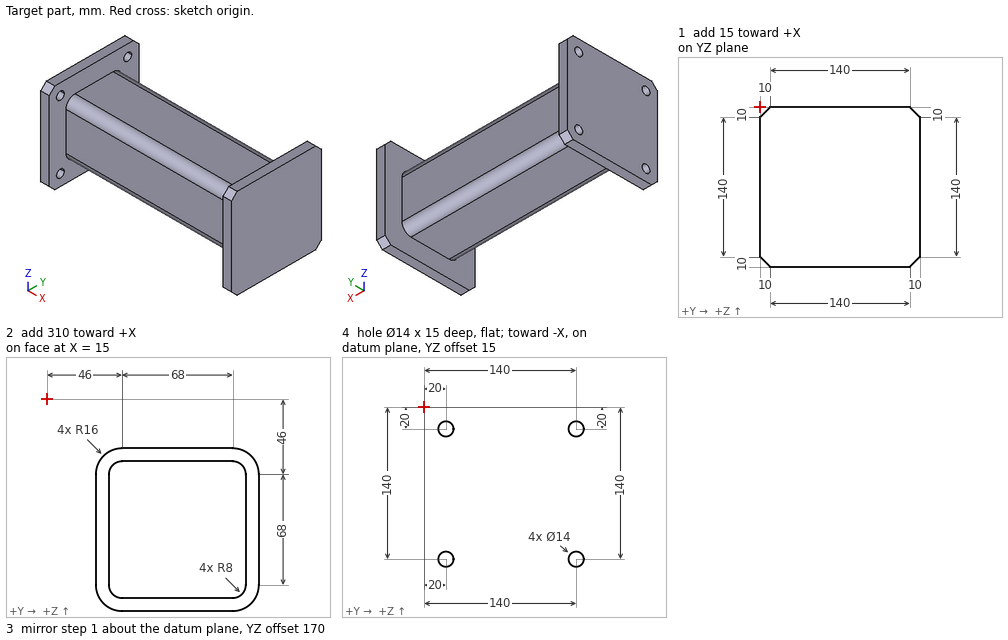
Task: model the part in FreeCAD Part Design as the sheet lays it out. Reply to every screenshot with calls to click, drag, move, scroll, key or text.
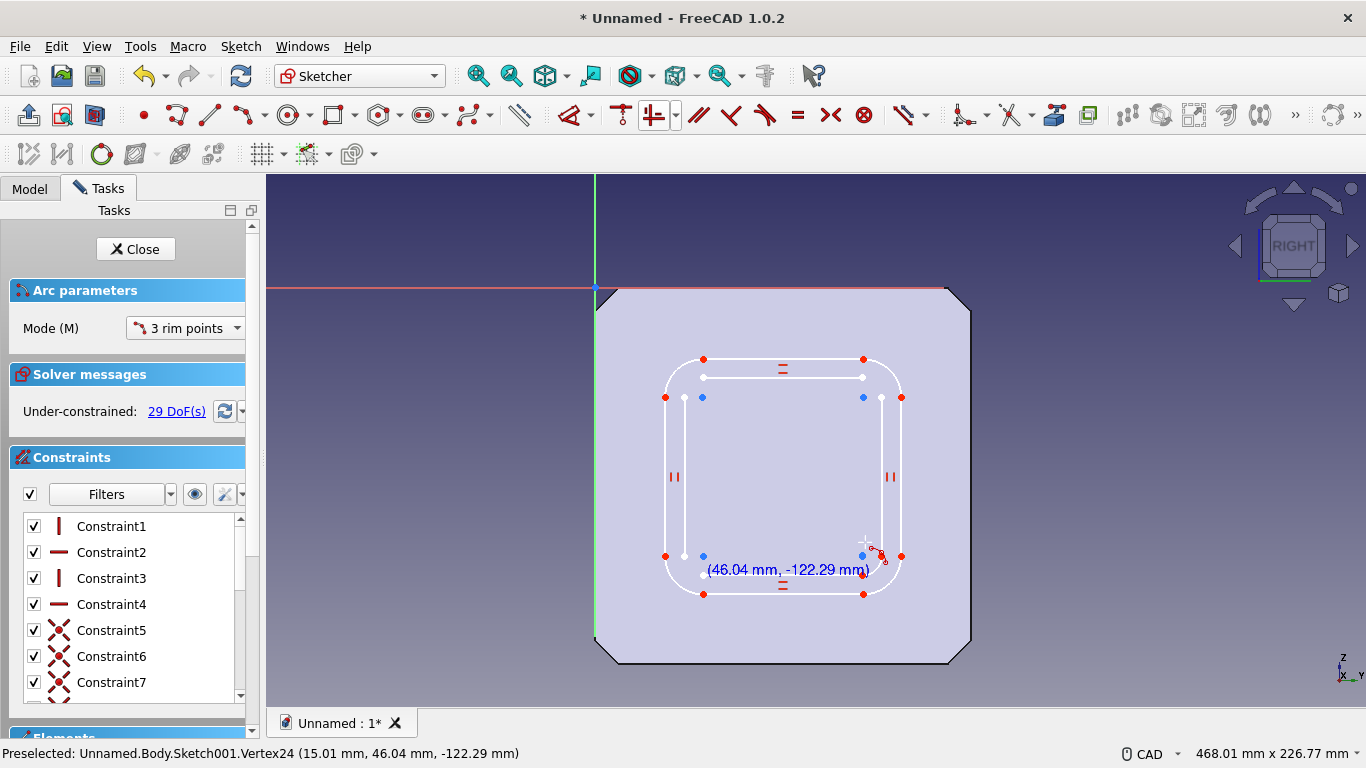
click(685, 557)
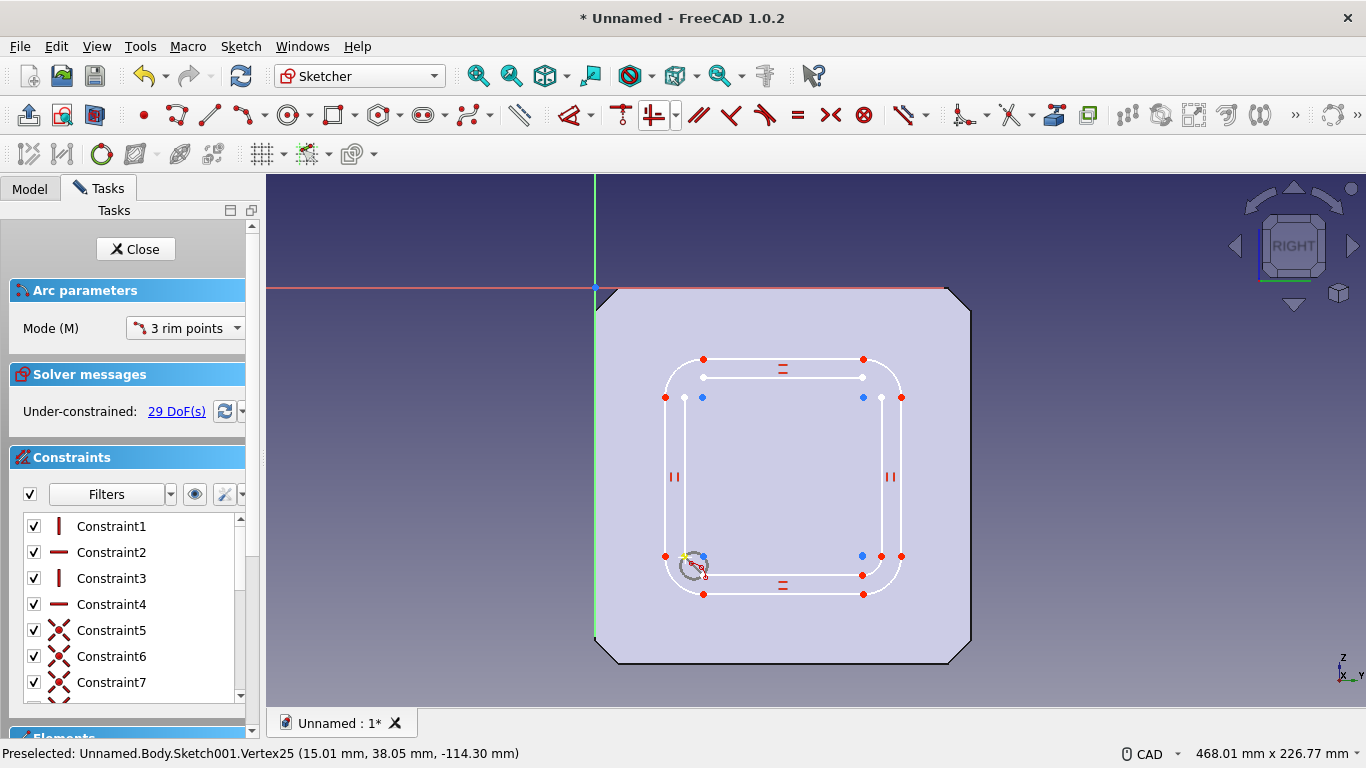
scroll(690, 569, up, 6)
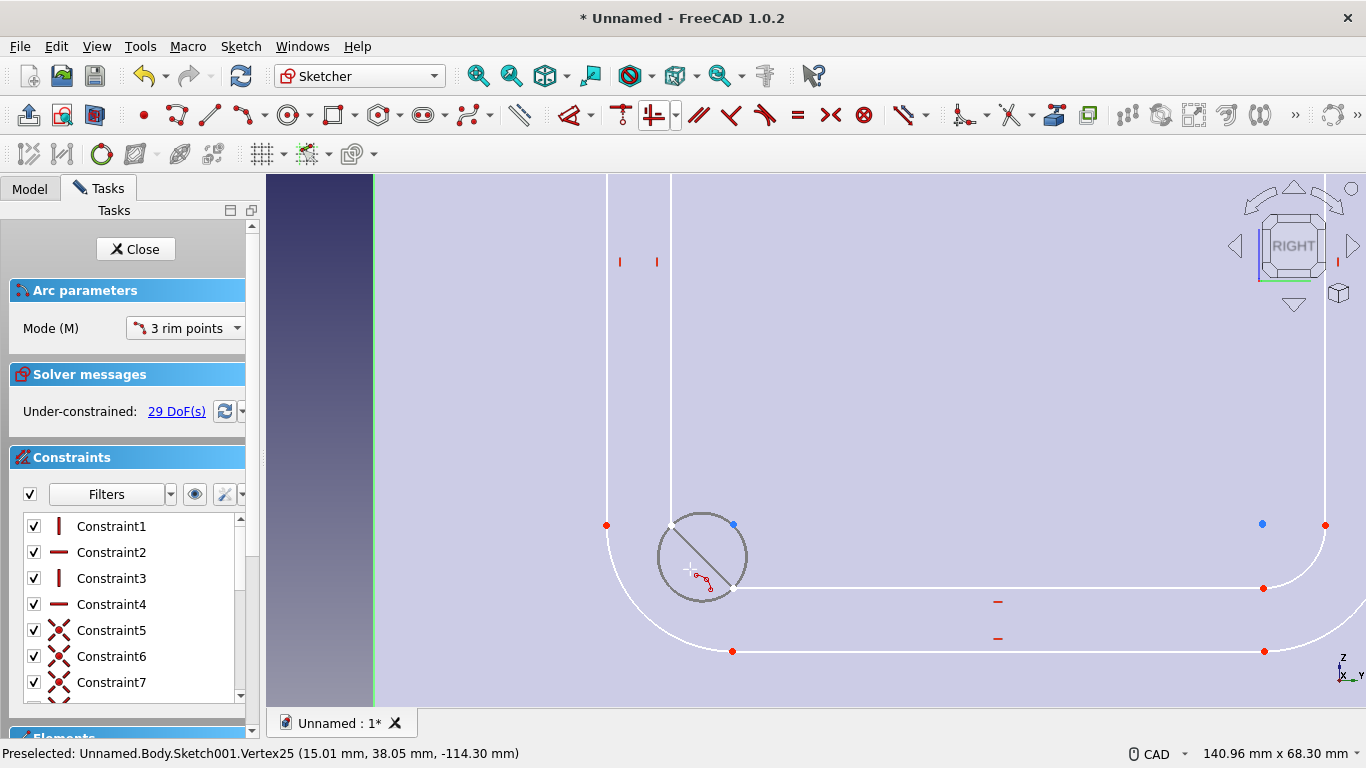
click(689, 568)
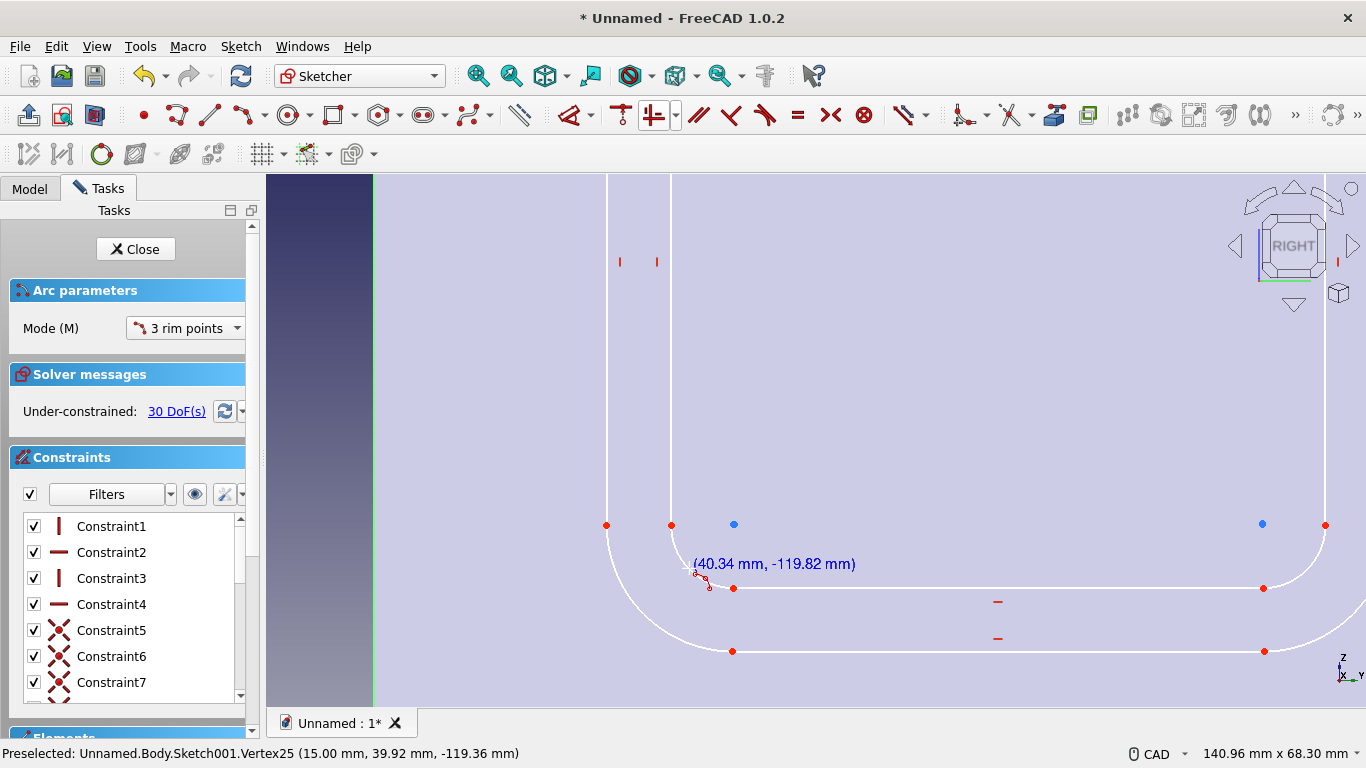
scroll(690, 570, down, 6)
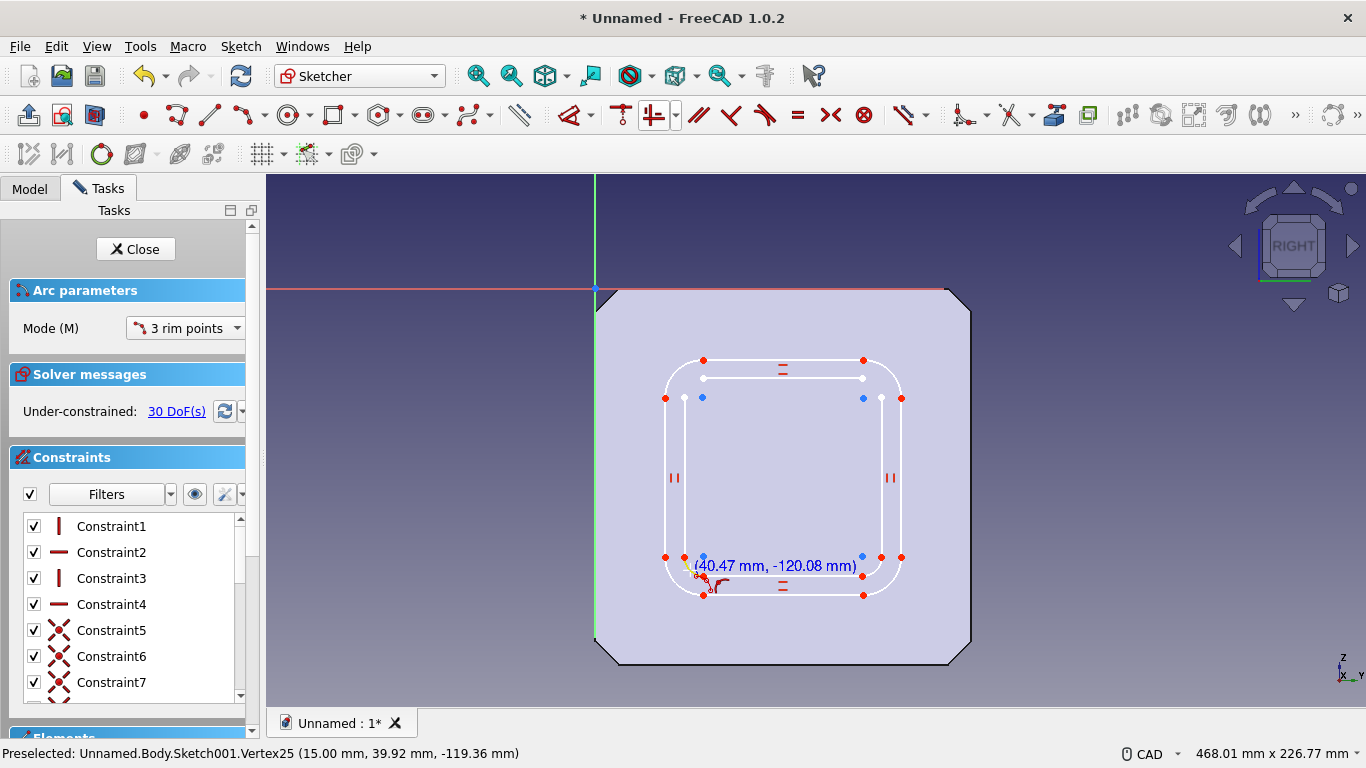
click(685, 398)
click(703, 378)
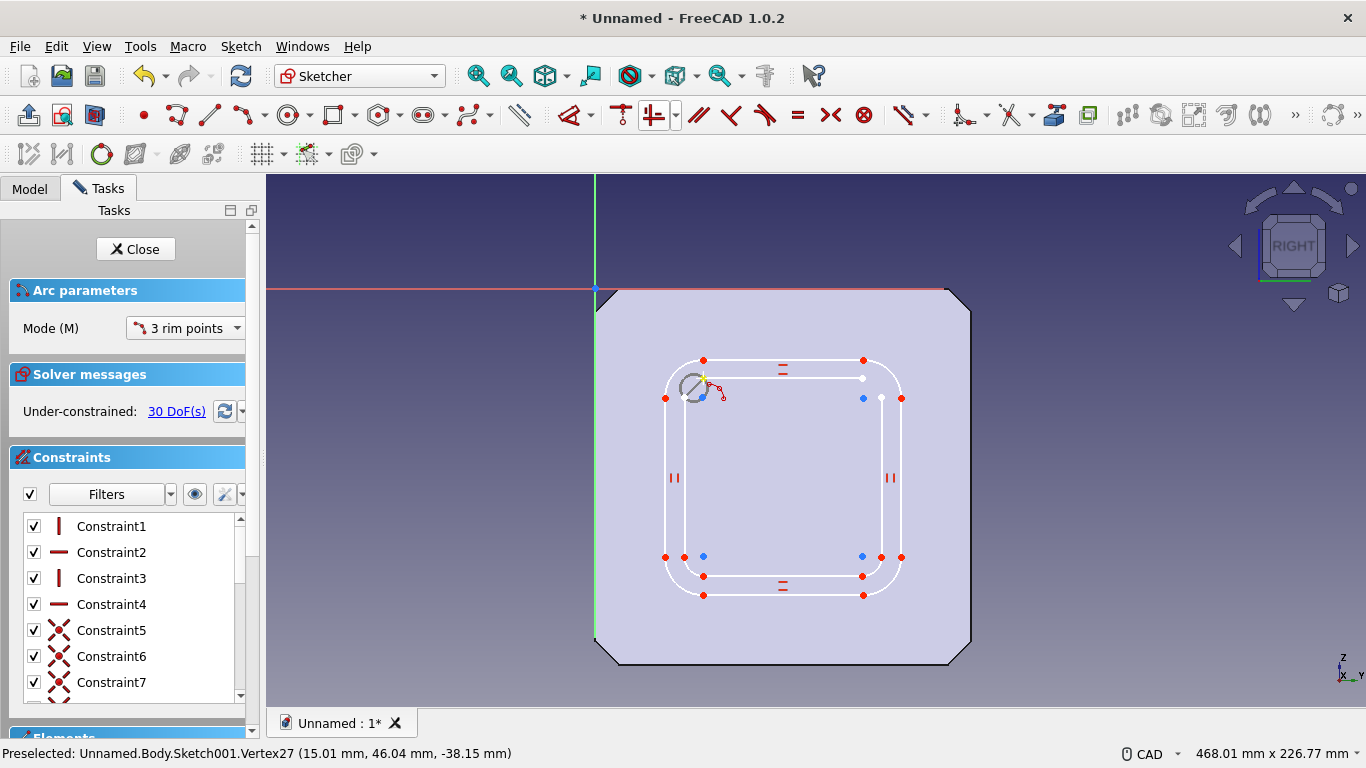
scroll(690, 383, up, 6)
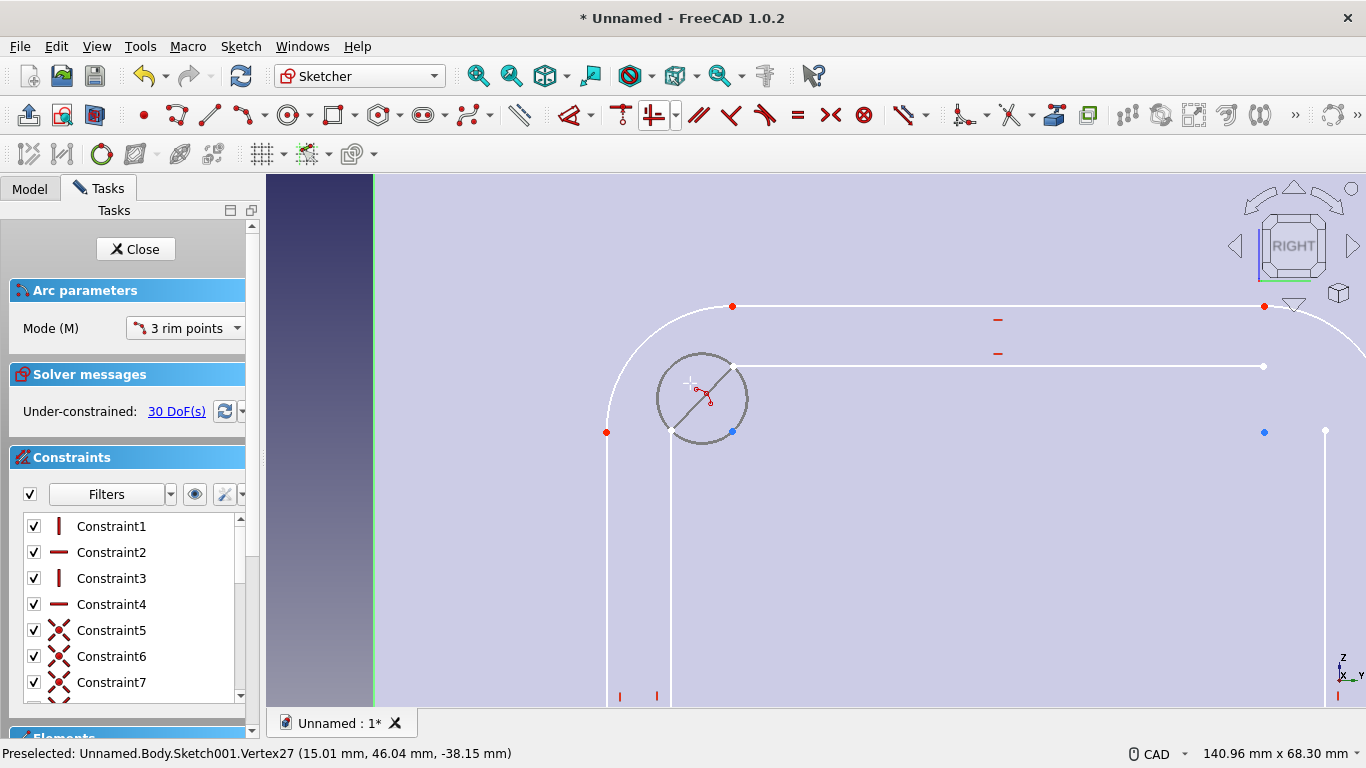
click(689, 383)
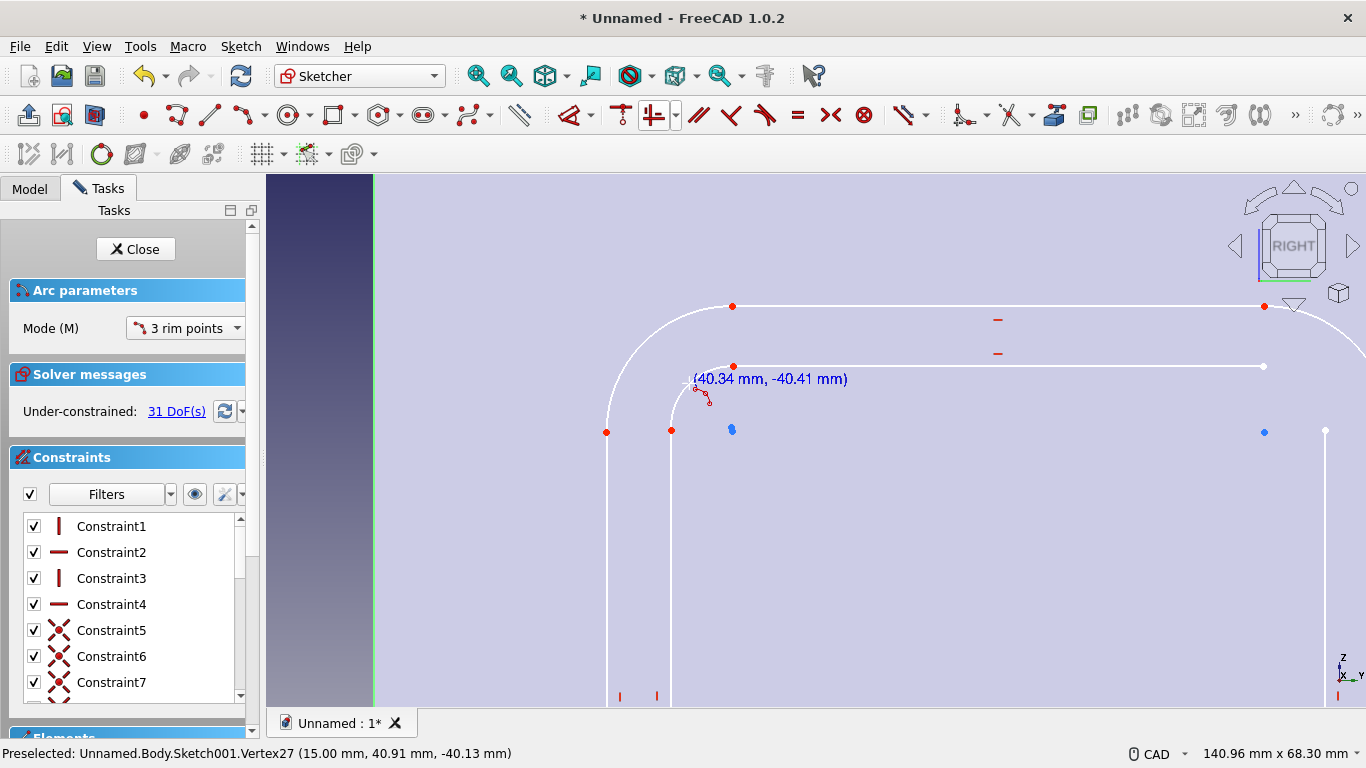
scroll(690, 382, down, 6)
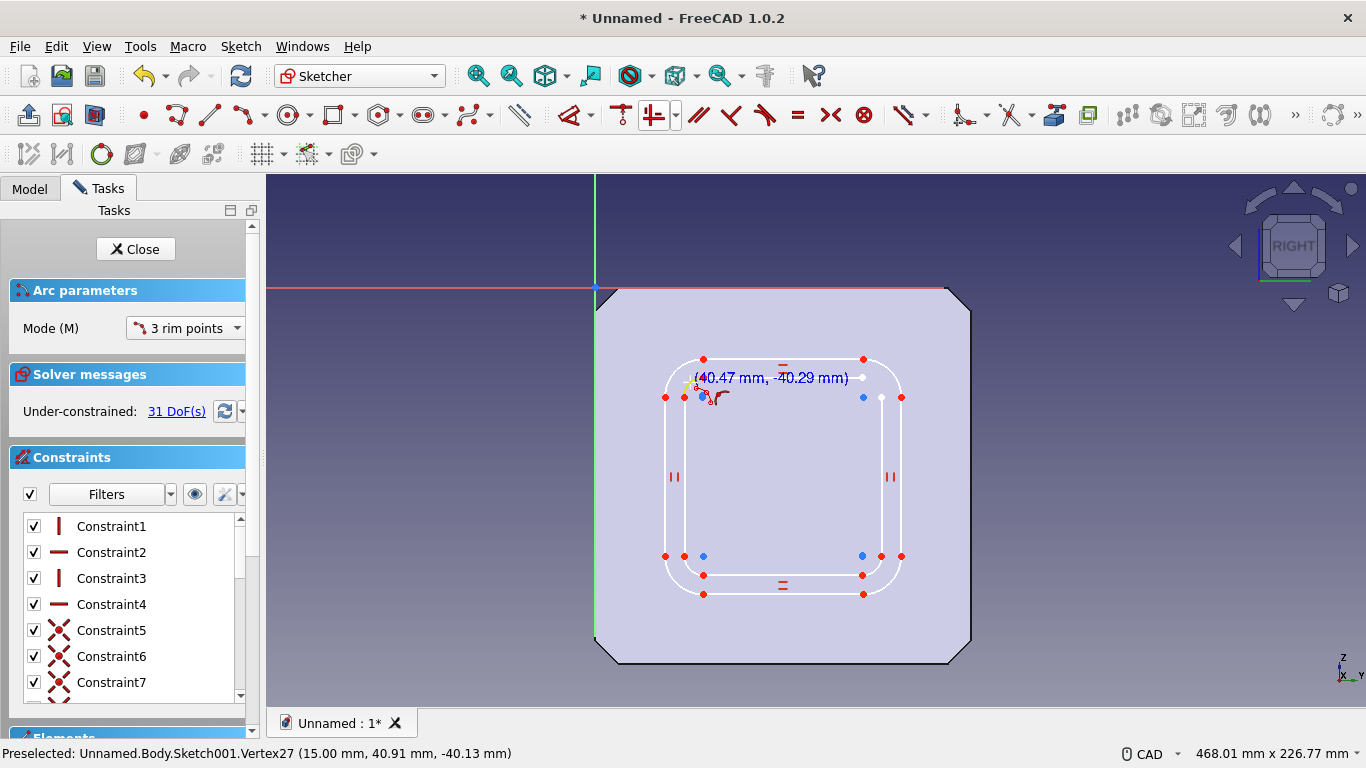
click(863, 378)
click(882, 397)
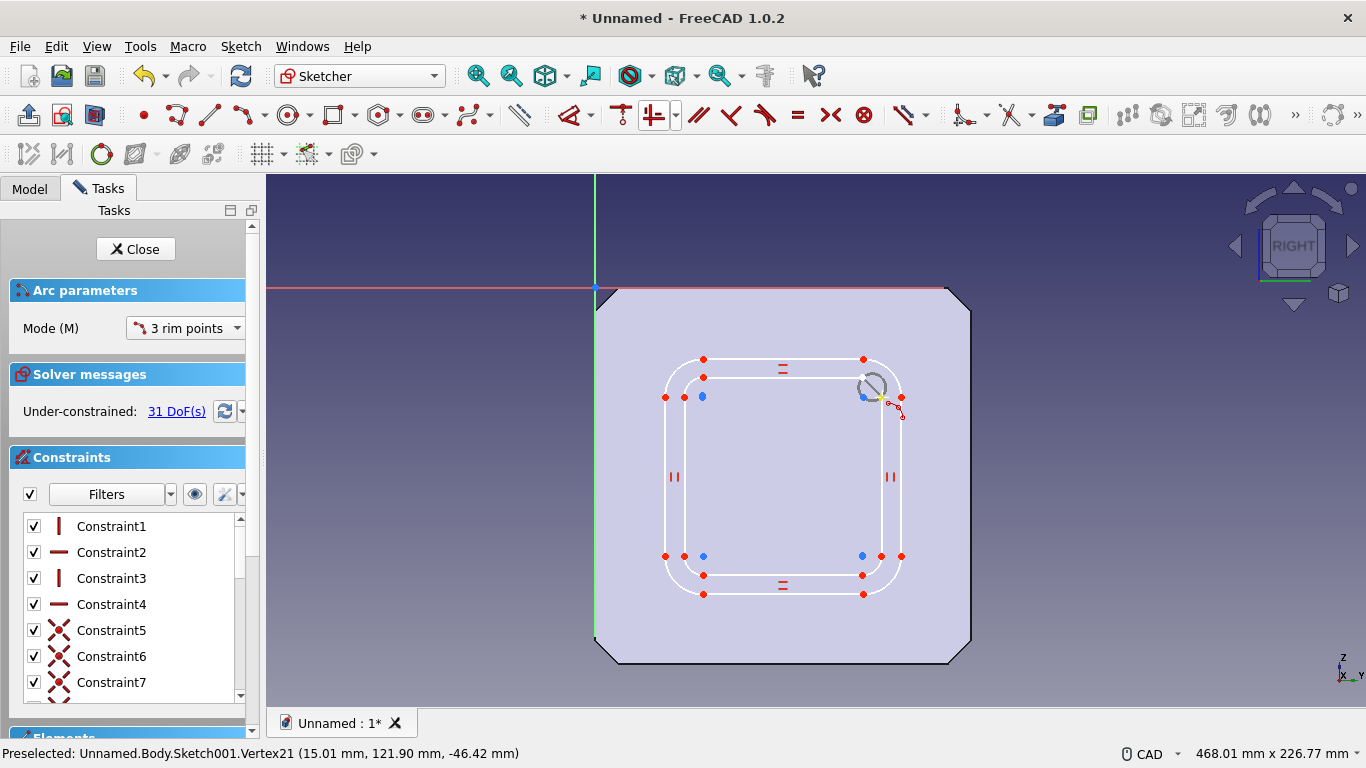
scroll(876, 383, up, 6)